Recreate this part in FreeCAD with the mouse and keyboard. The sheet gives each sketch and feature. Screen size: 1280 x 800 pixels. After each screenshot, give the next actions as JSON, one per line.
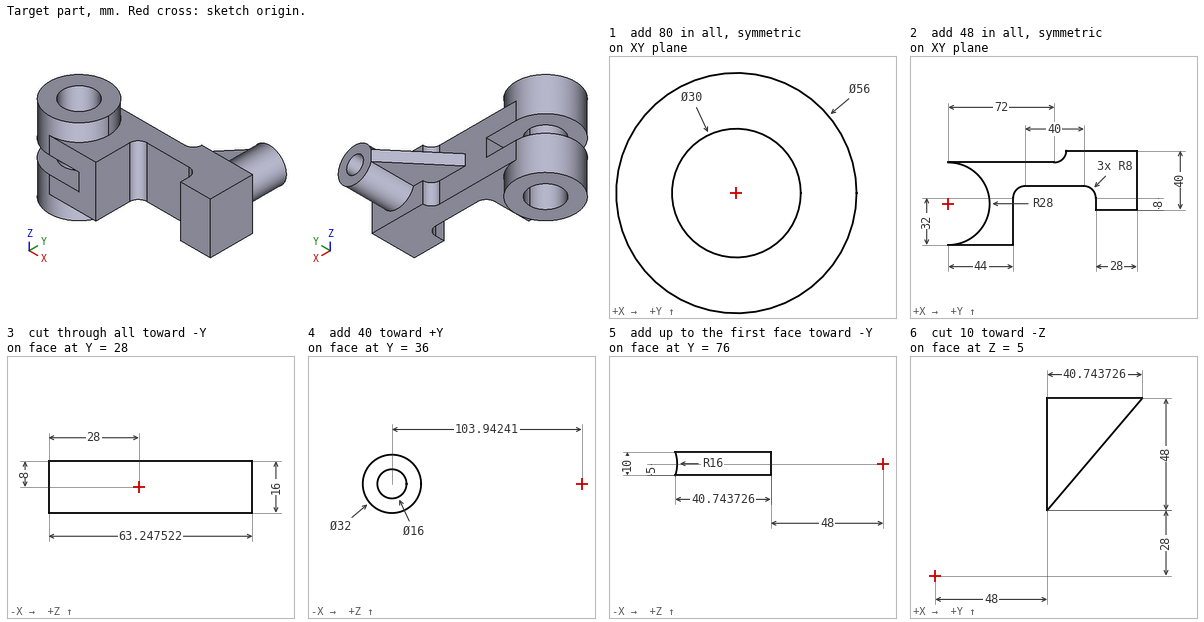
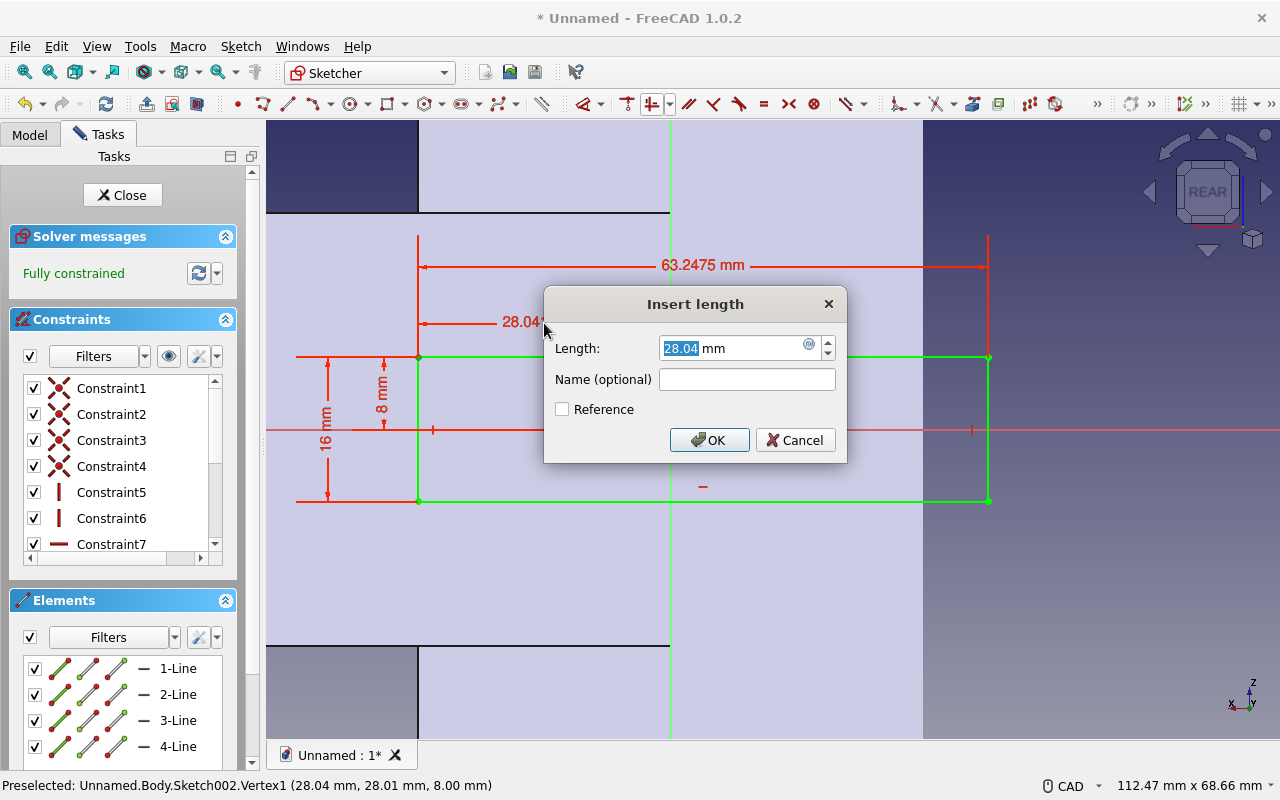
{"action": "type", "text": "28"}
{"action": "key", "text": "Return"}
{"action": "key", "text": "Escape"}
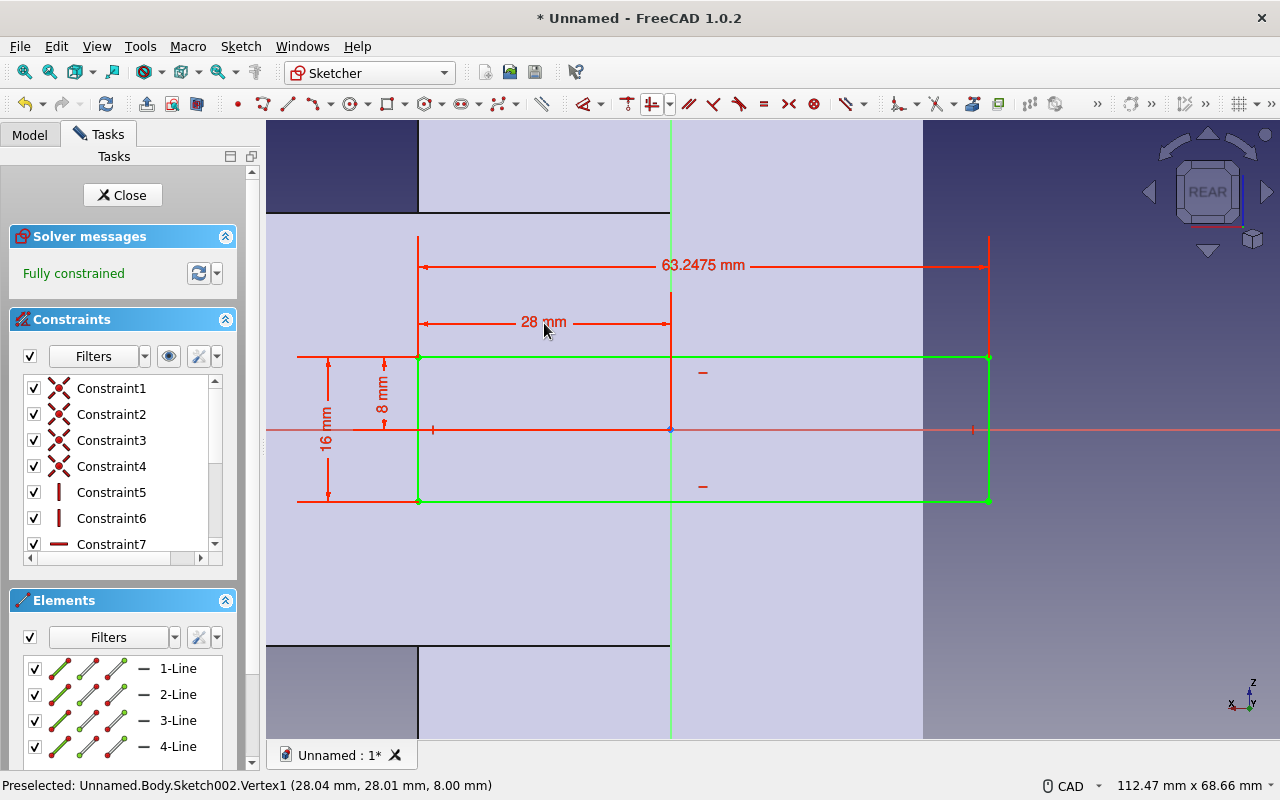
{"action": "left_click", "coordinate": [123, 195]}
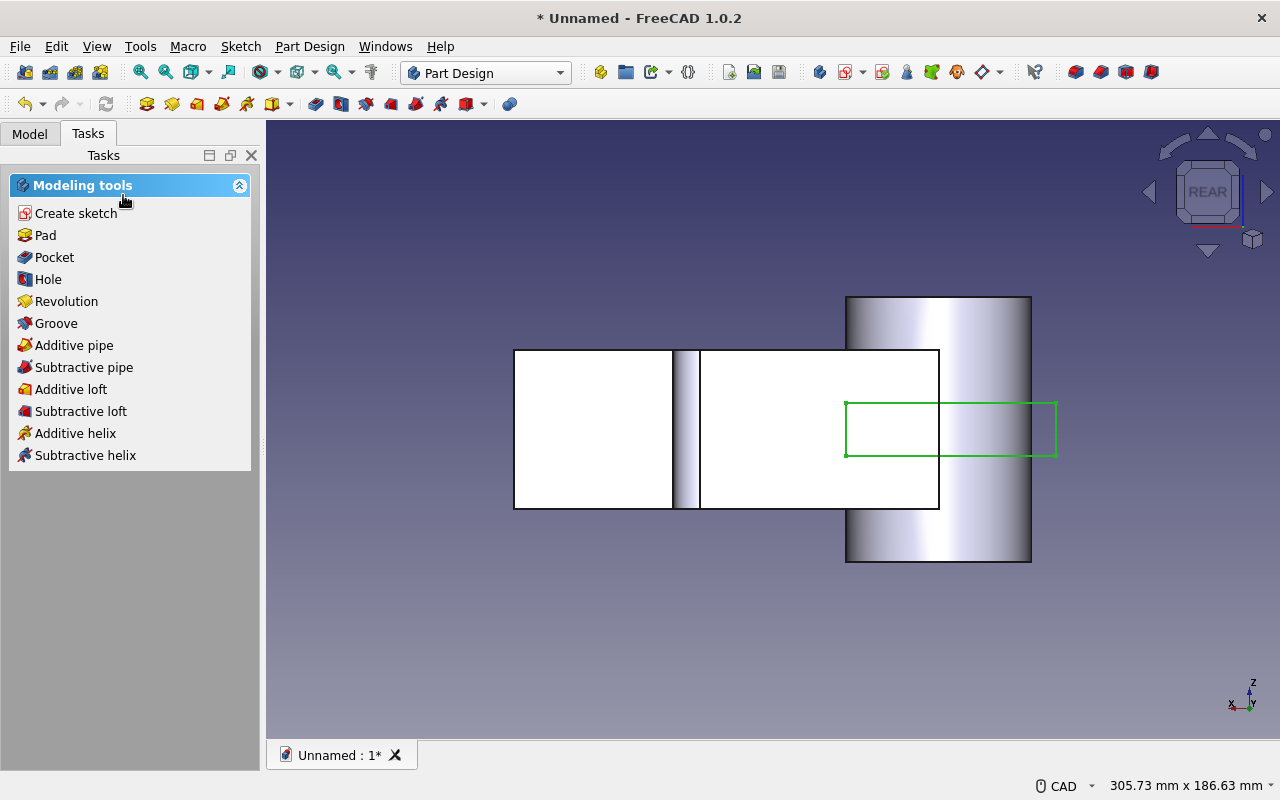
{"action": "left_click", "coordinate": [316, 104]}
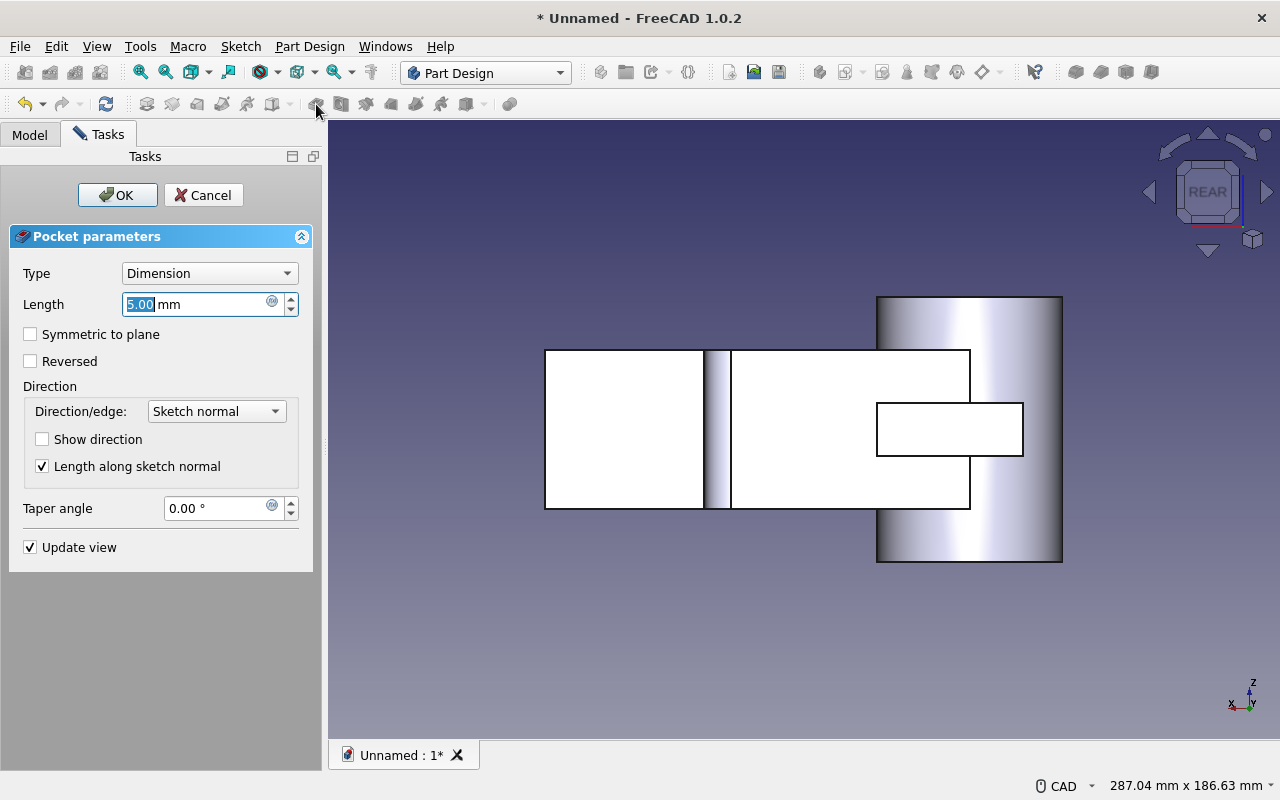
{"action": "left_click", "coordinate": [210, 274]}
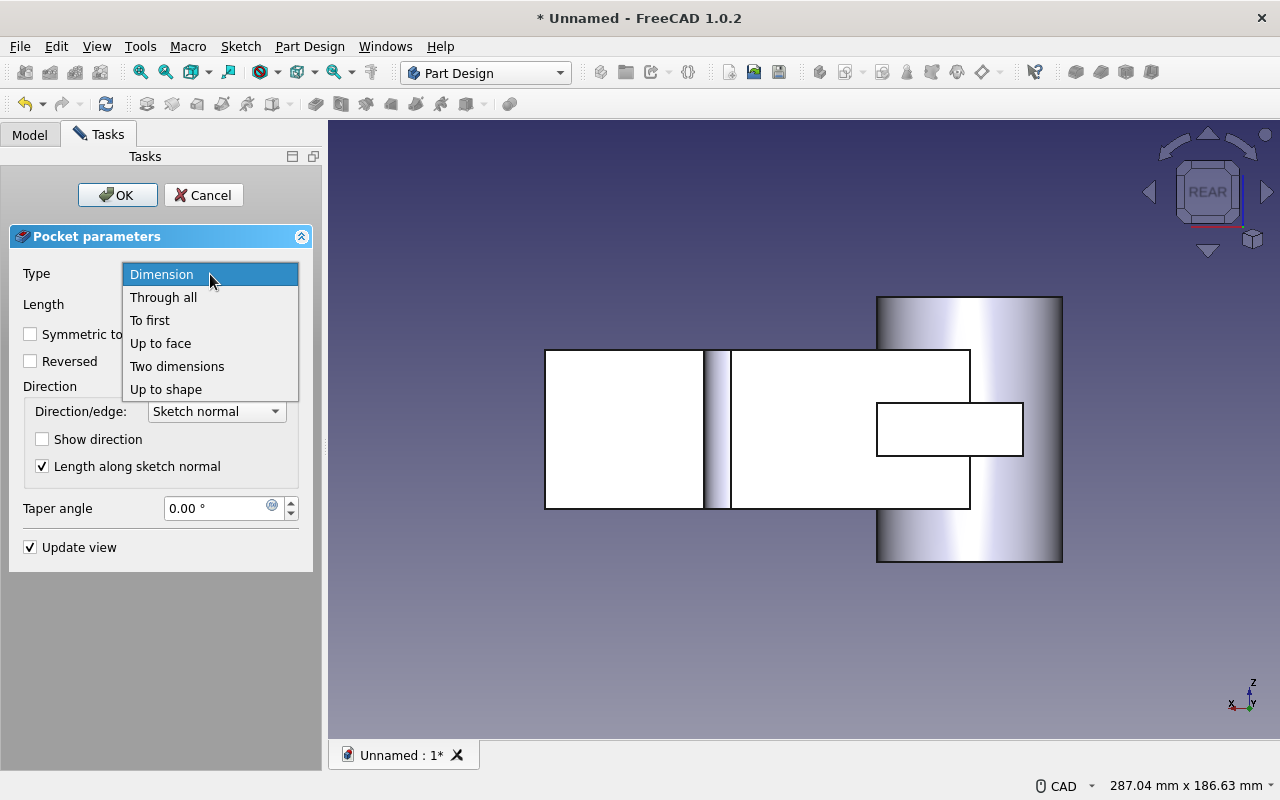
{"action": "left_click", "coordinate": [208, 298]}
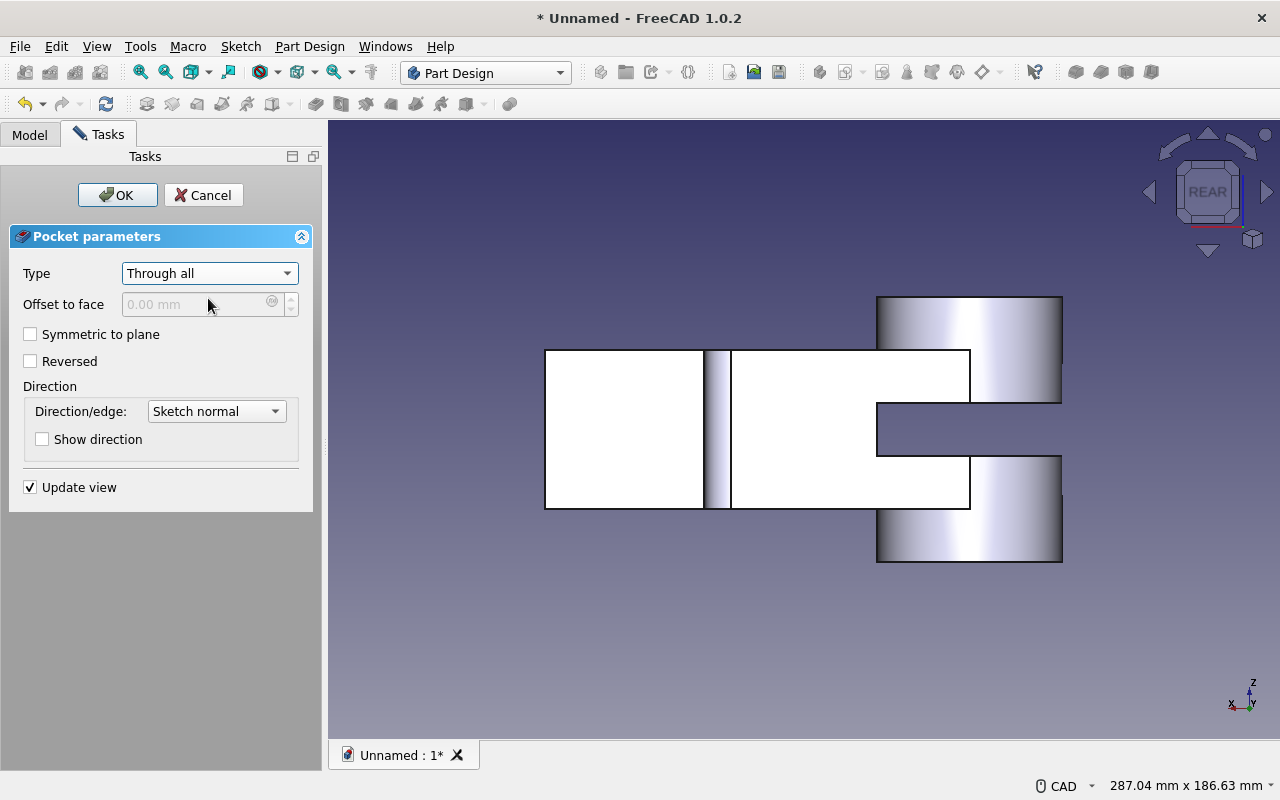
{"action": "left_click", "coordinate": [118, 195]}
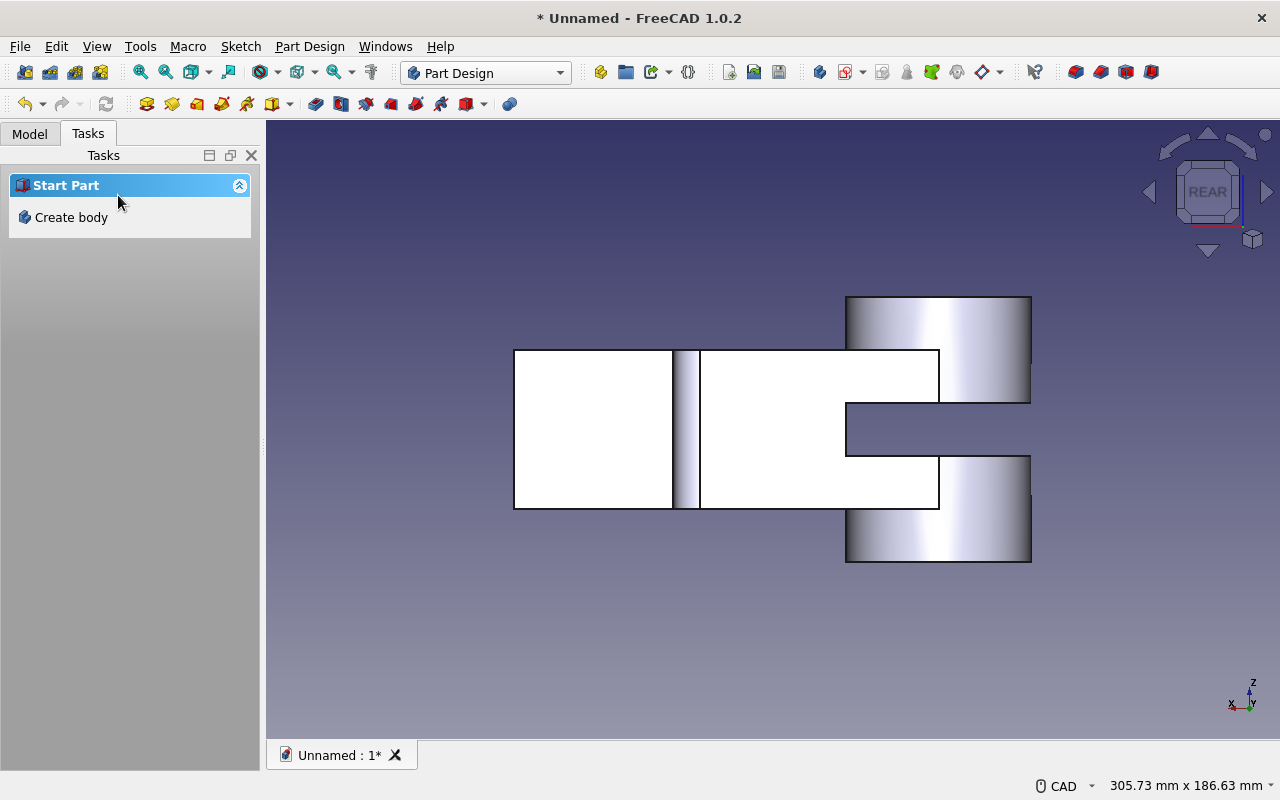
{"action": "left_click", "coordinate": [594, 428]}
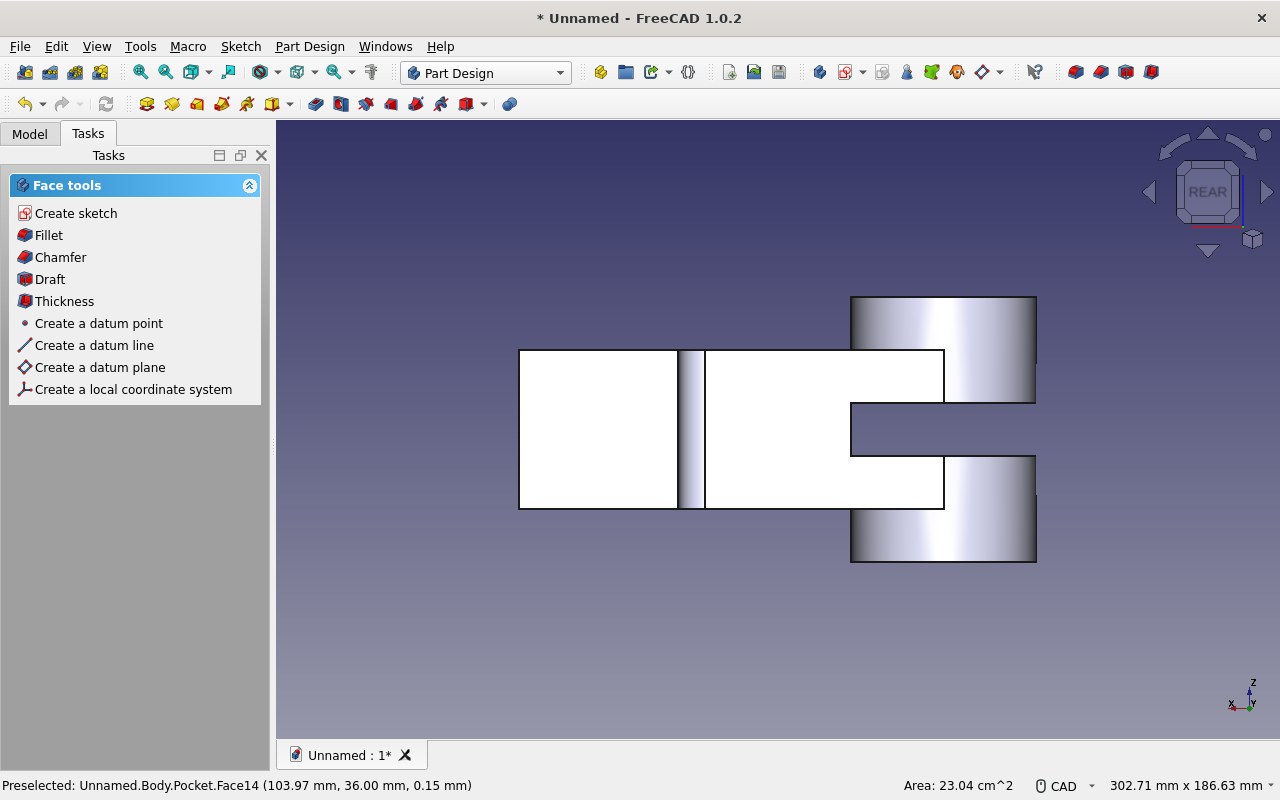
{"action": "left_click", "coordinate": [844, 72]}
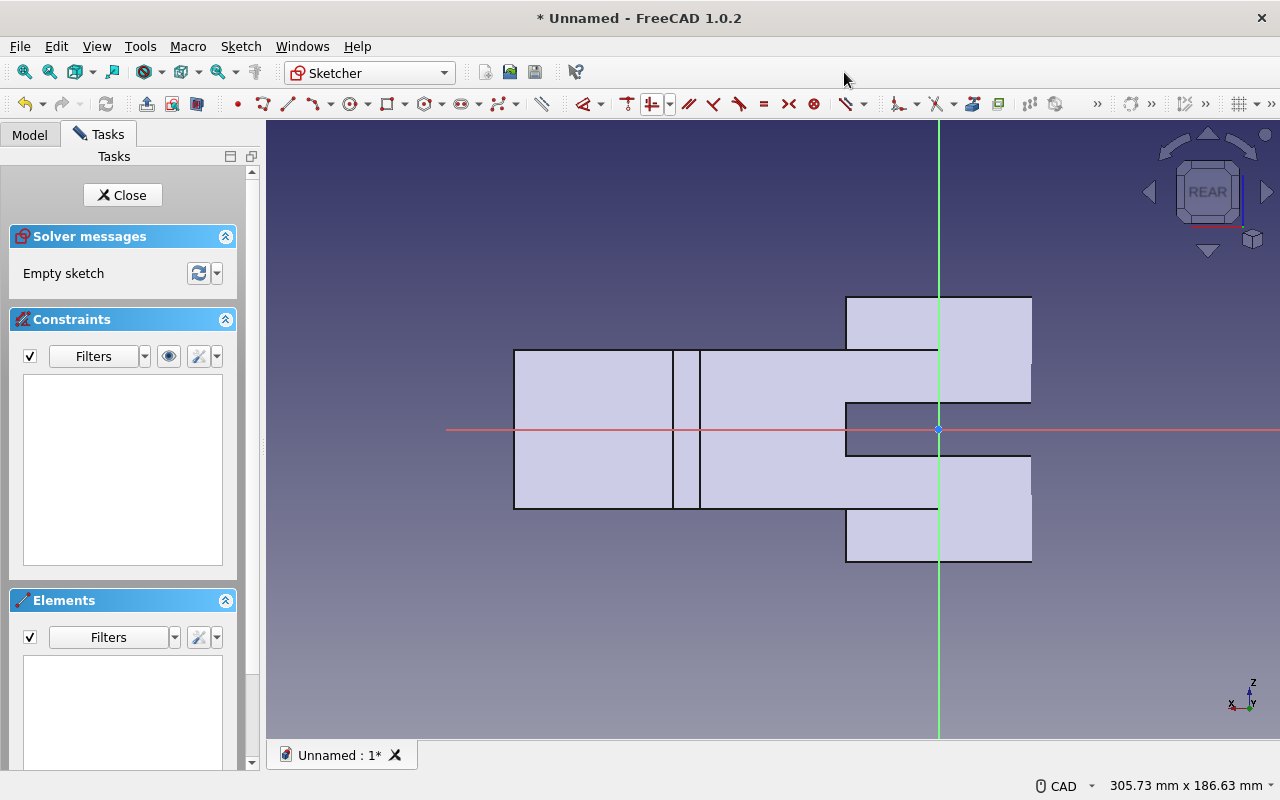
{"action": "scroll", "coordinate": [558, 430], "scroll_direction": "up", "scroll_amount": 7}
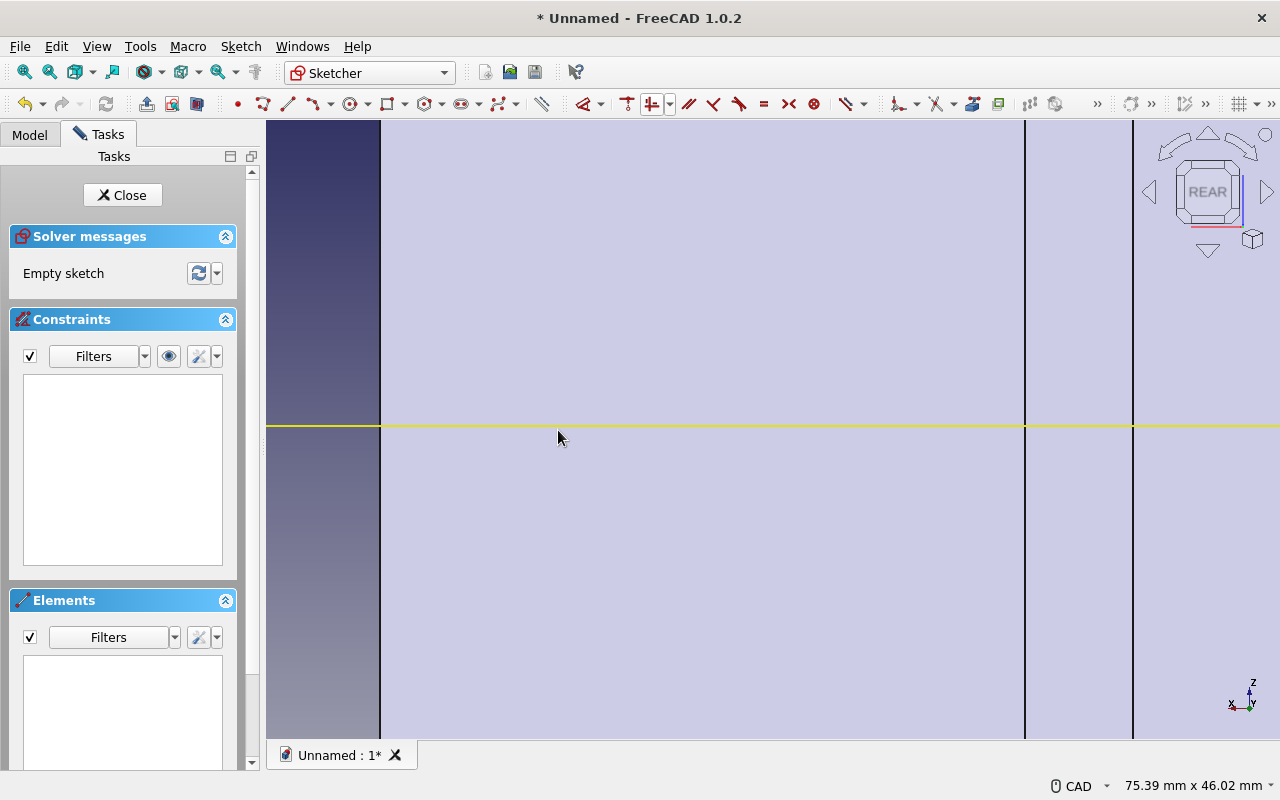
{"action": "left_click", "coordinate": [350, 104]}